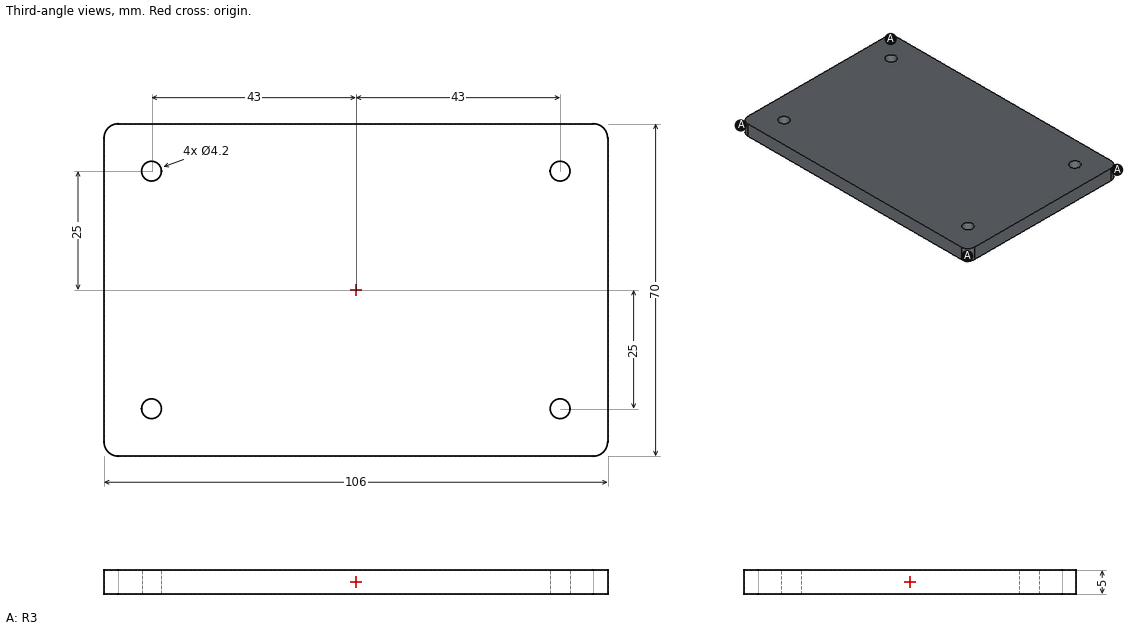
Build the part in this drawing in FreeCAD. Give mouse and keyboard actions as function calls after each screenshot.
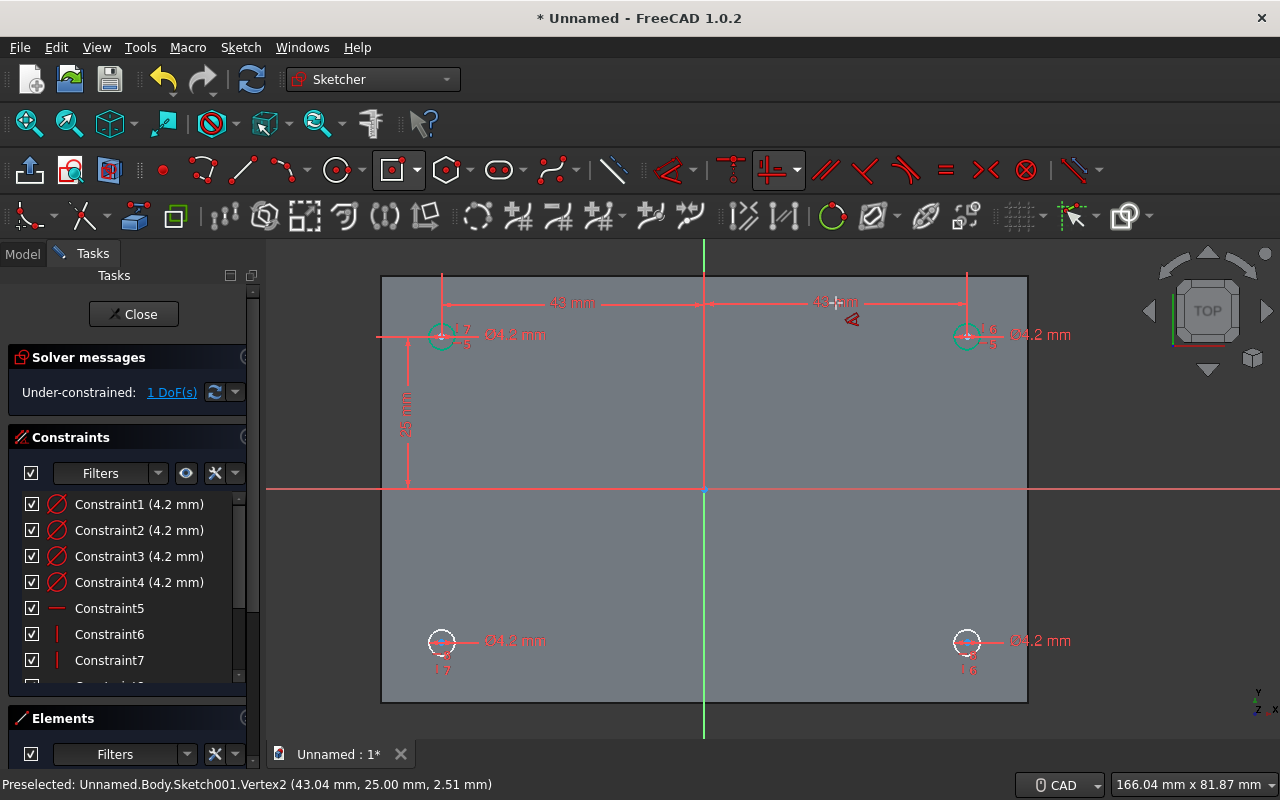
click(967, 643)
click(1001, 566)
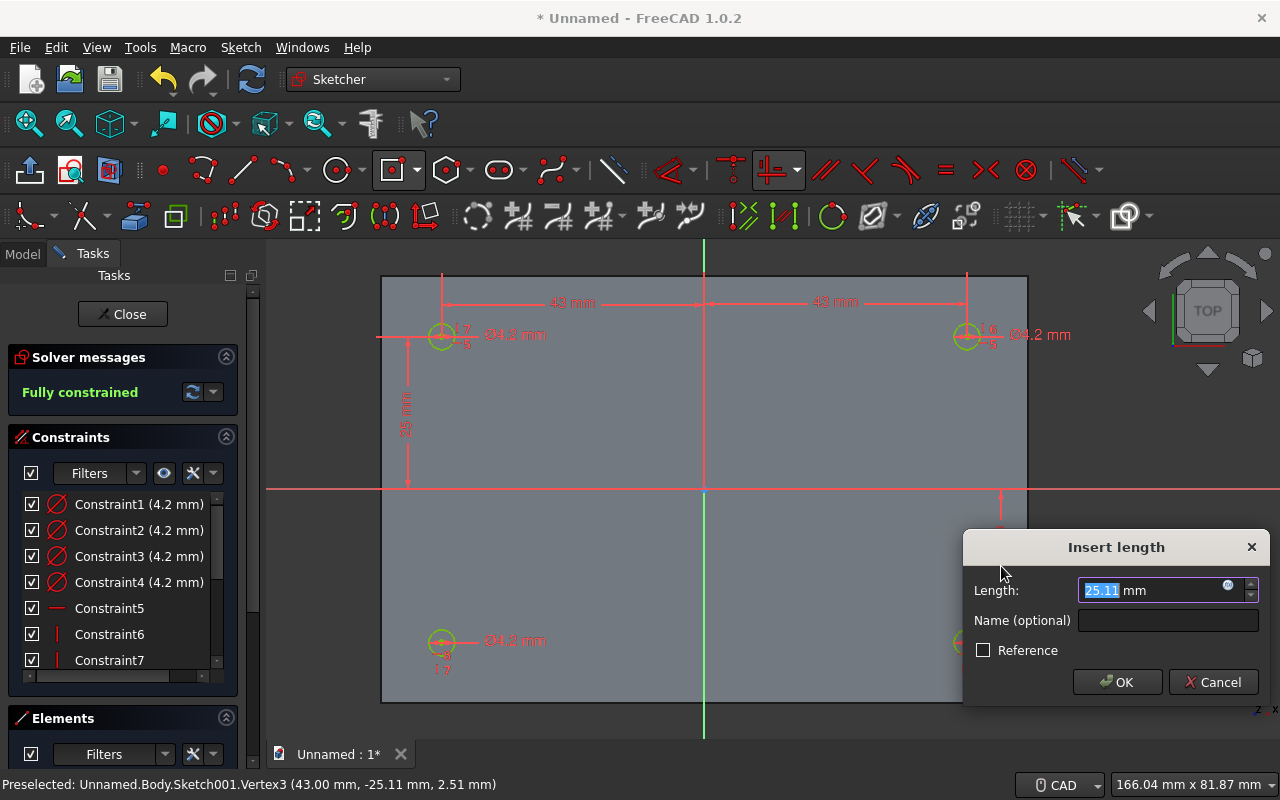
text(25)
key(Return)
key(Escape)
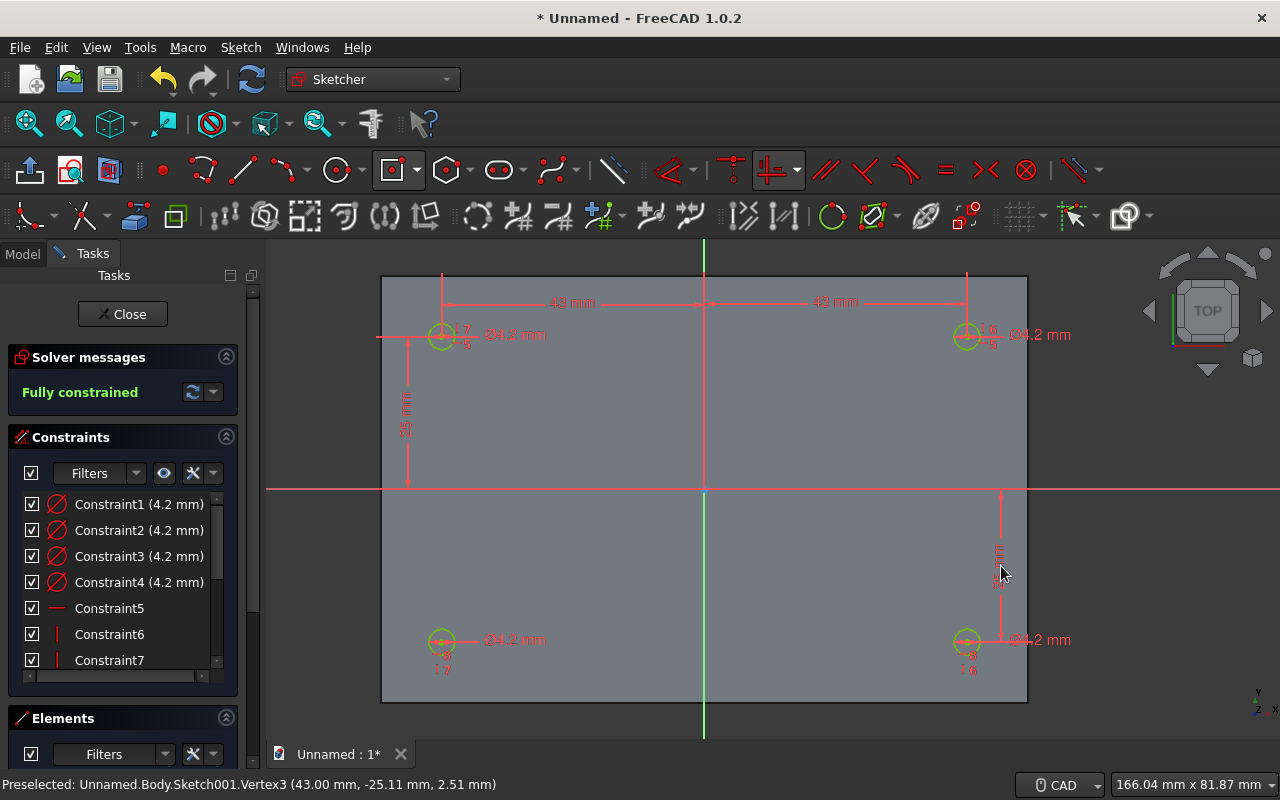
click(123, 314)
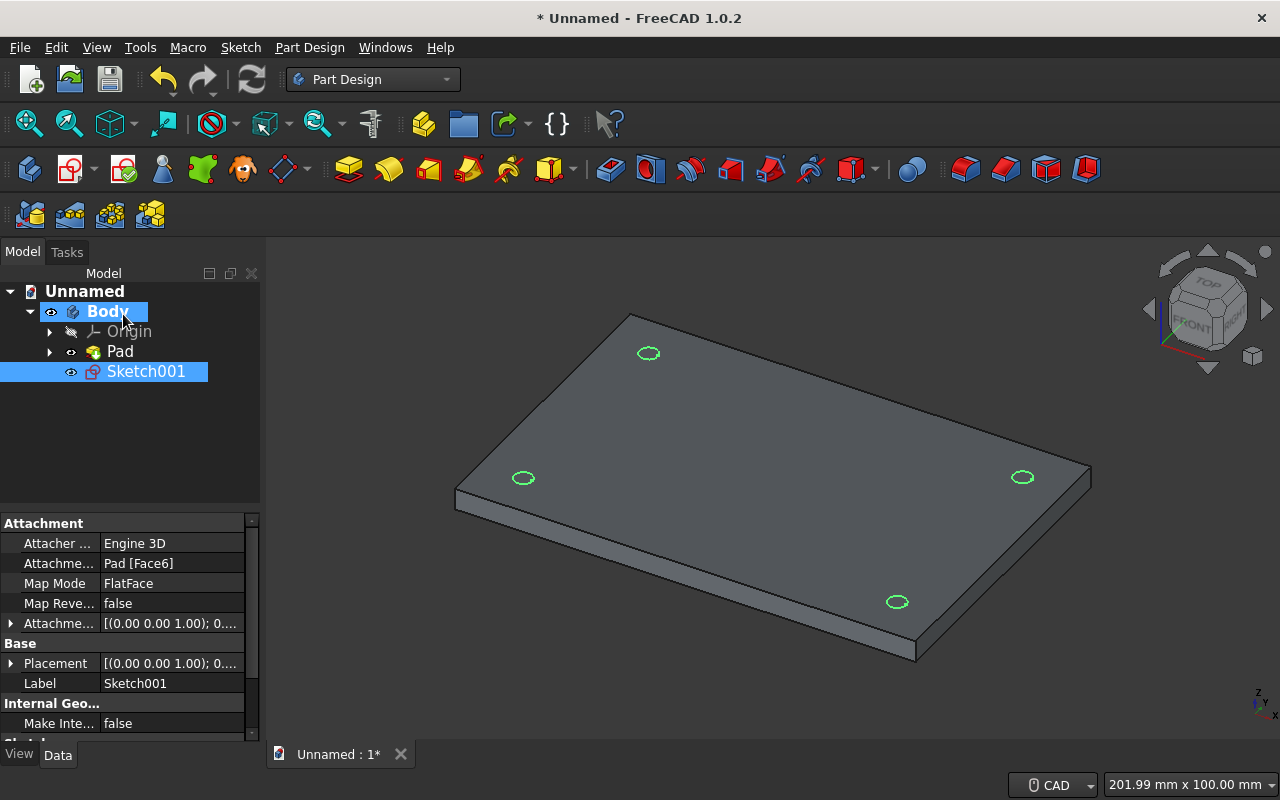
click(612, 170)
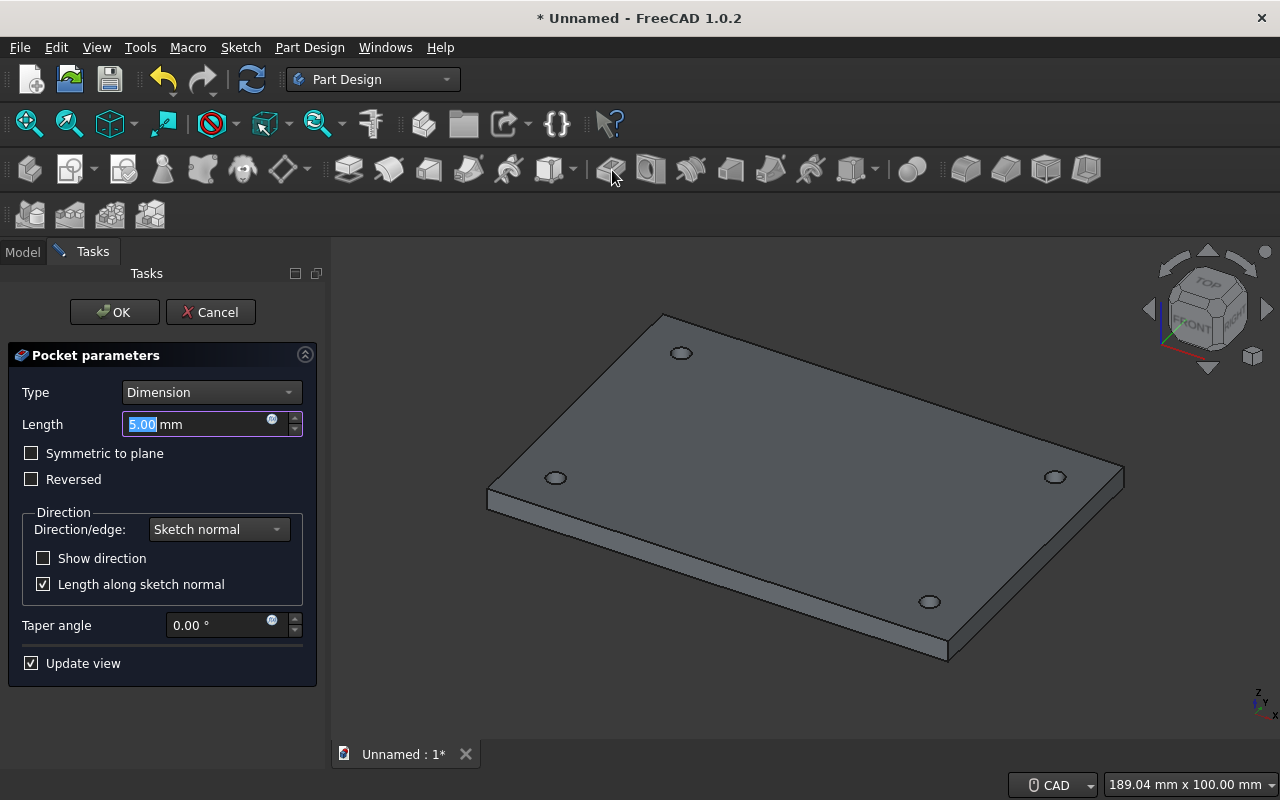
click(212, 392)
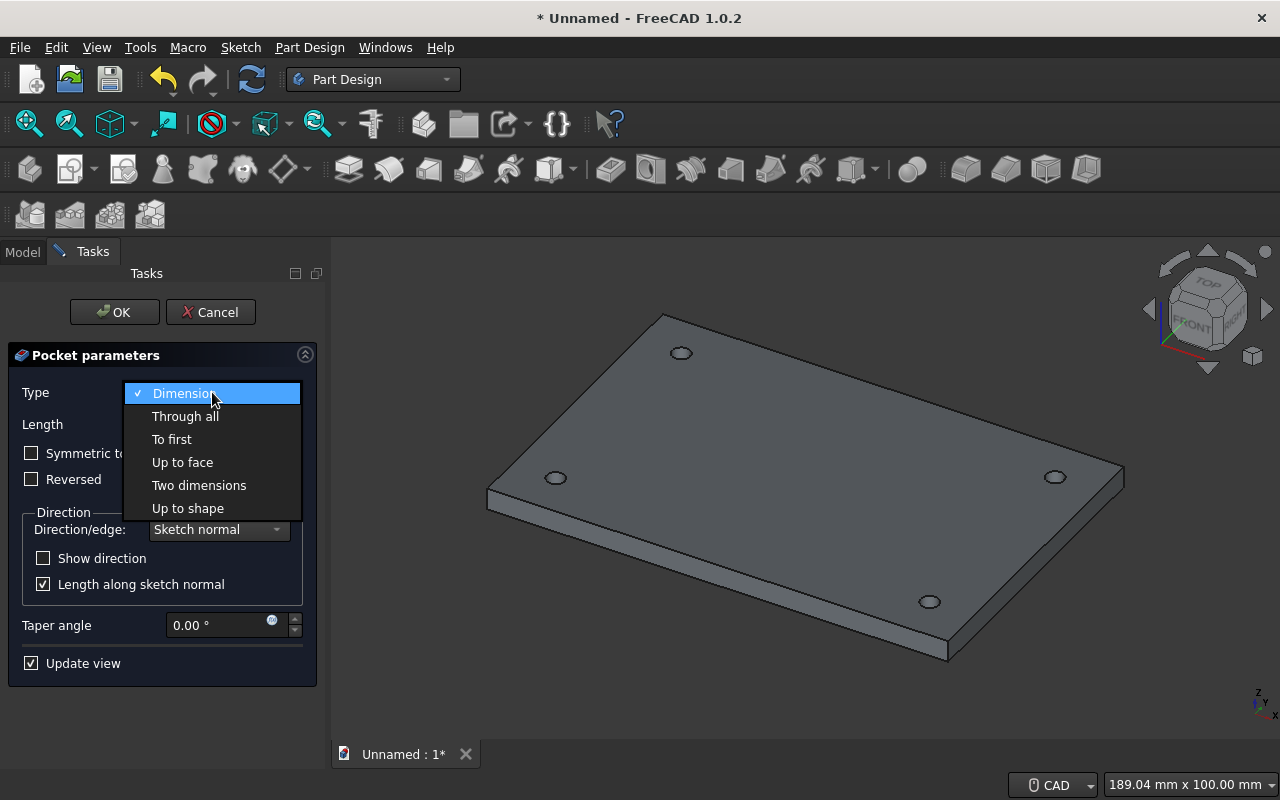
click(212, 416)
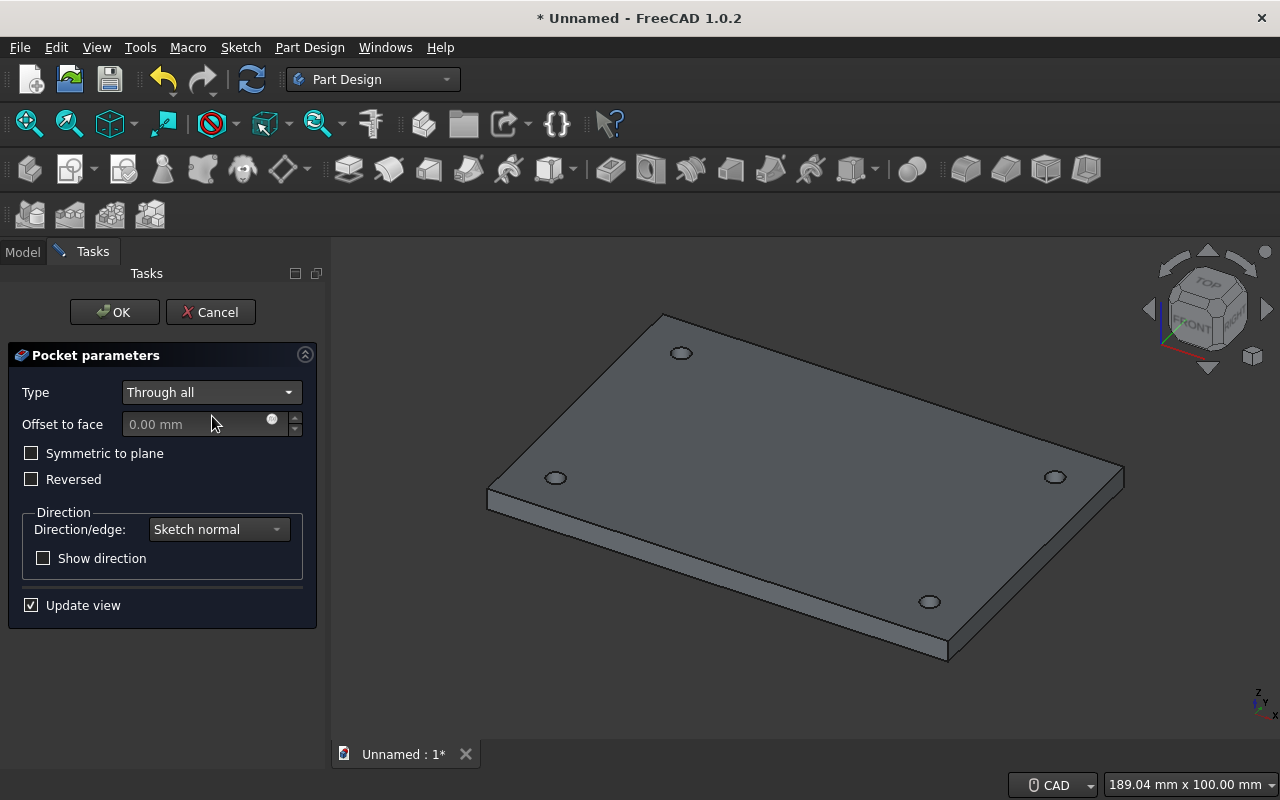
click(115, 312)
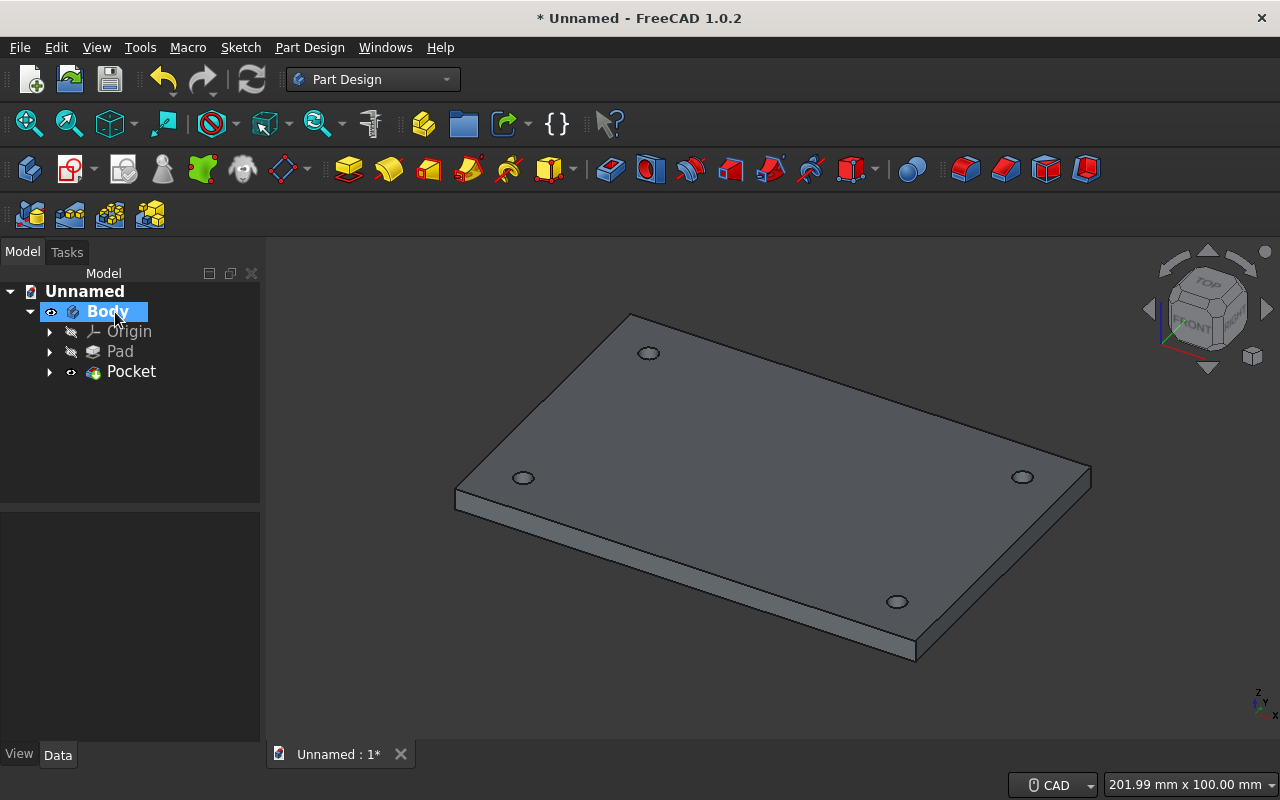
click(916, 651)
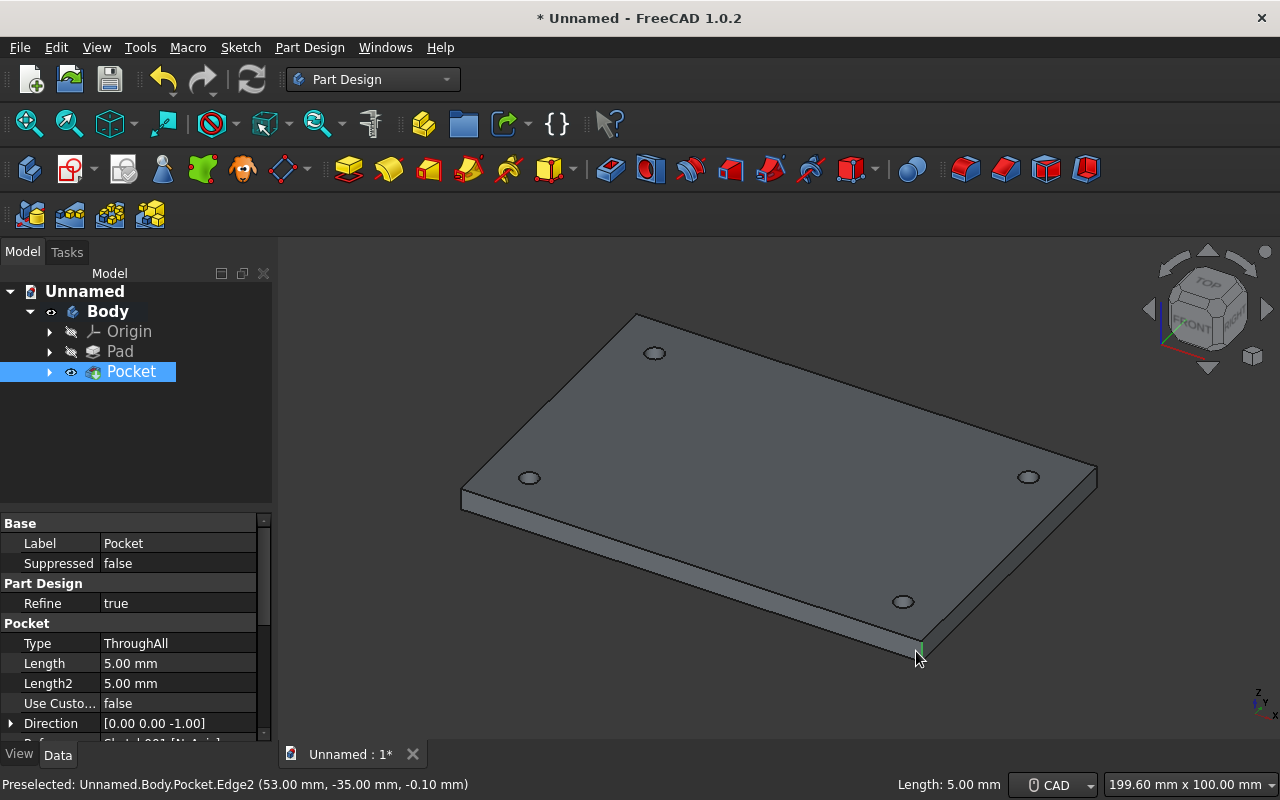
key(0)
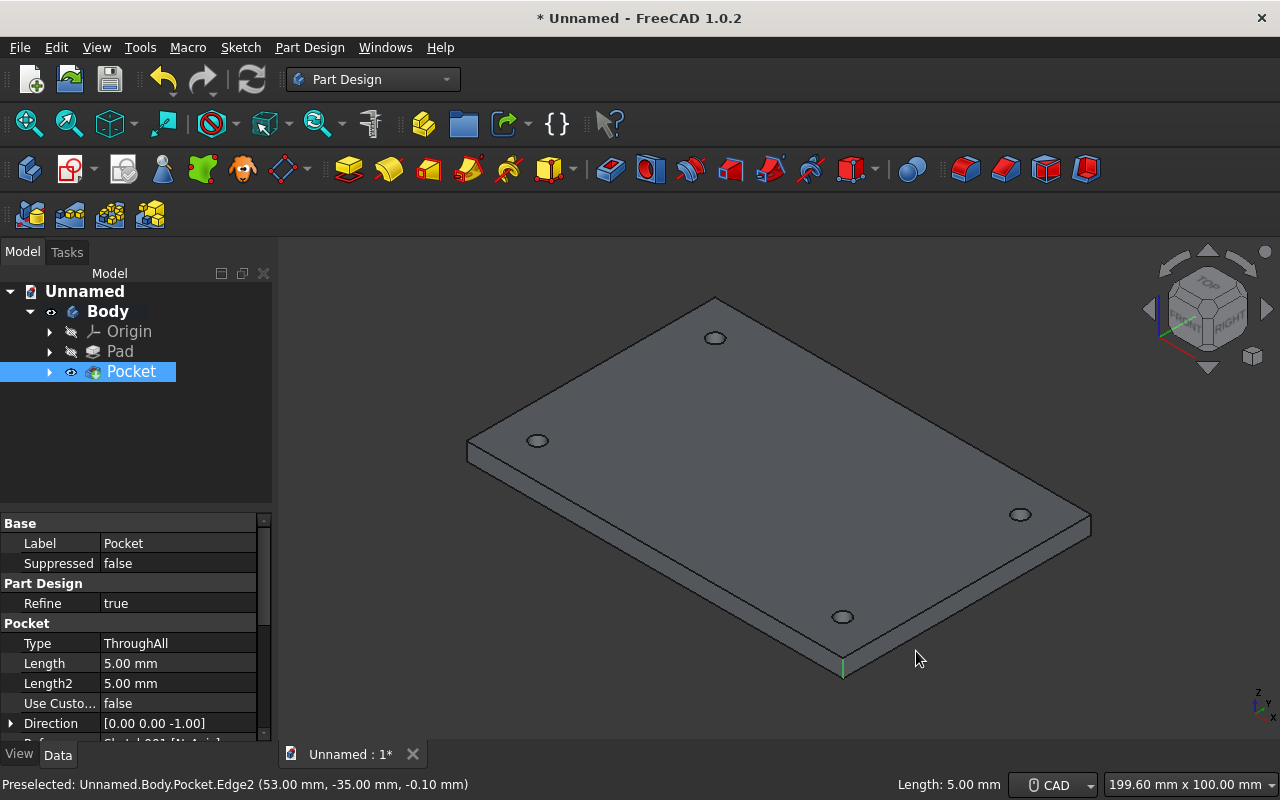
key(2)